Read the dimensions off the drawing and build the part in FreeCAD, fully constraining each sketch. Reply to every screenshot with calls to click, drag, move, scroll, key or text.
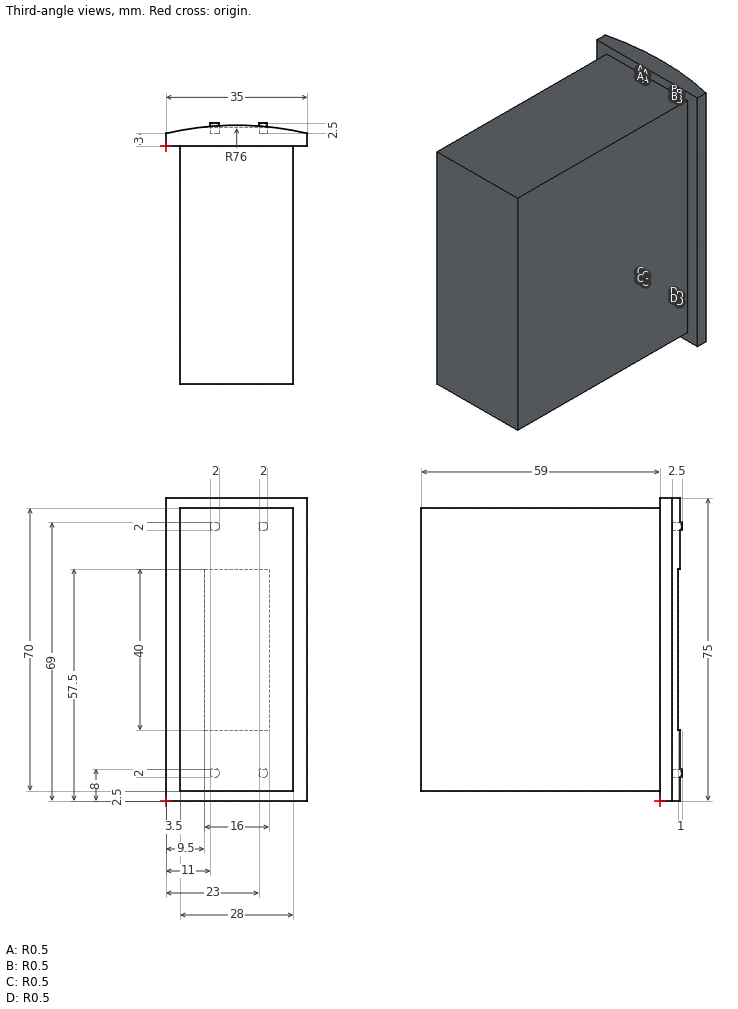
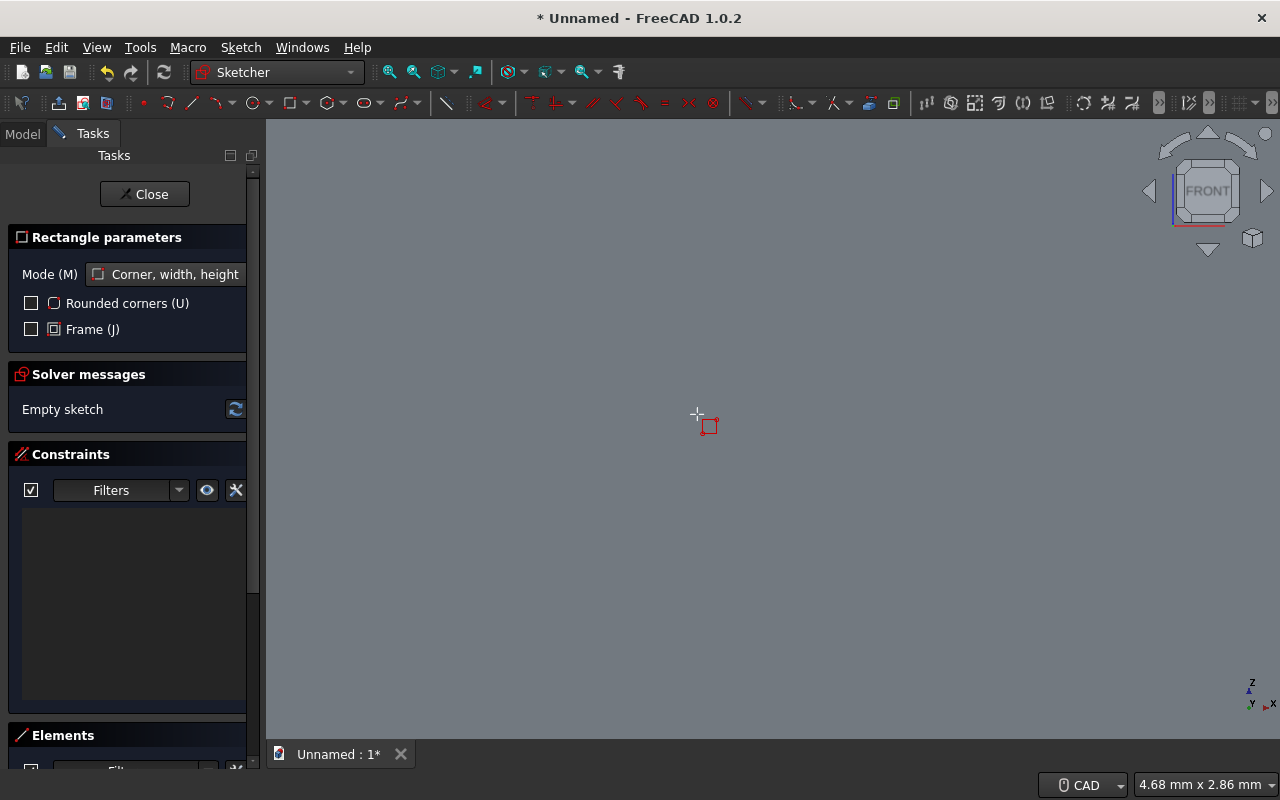
click(487, 212)
click(921, 645)
key(Escape)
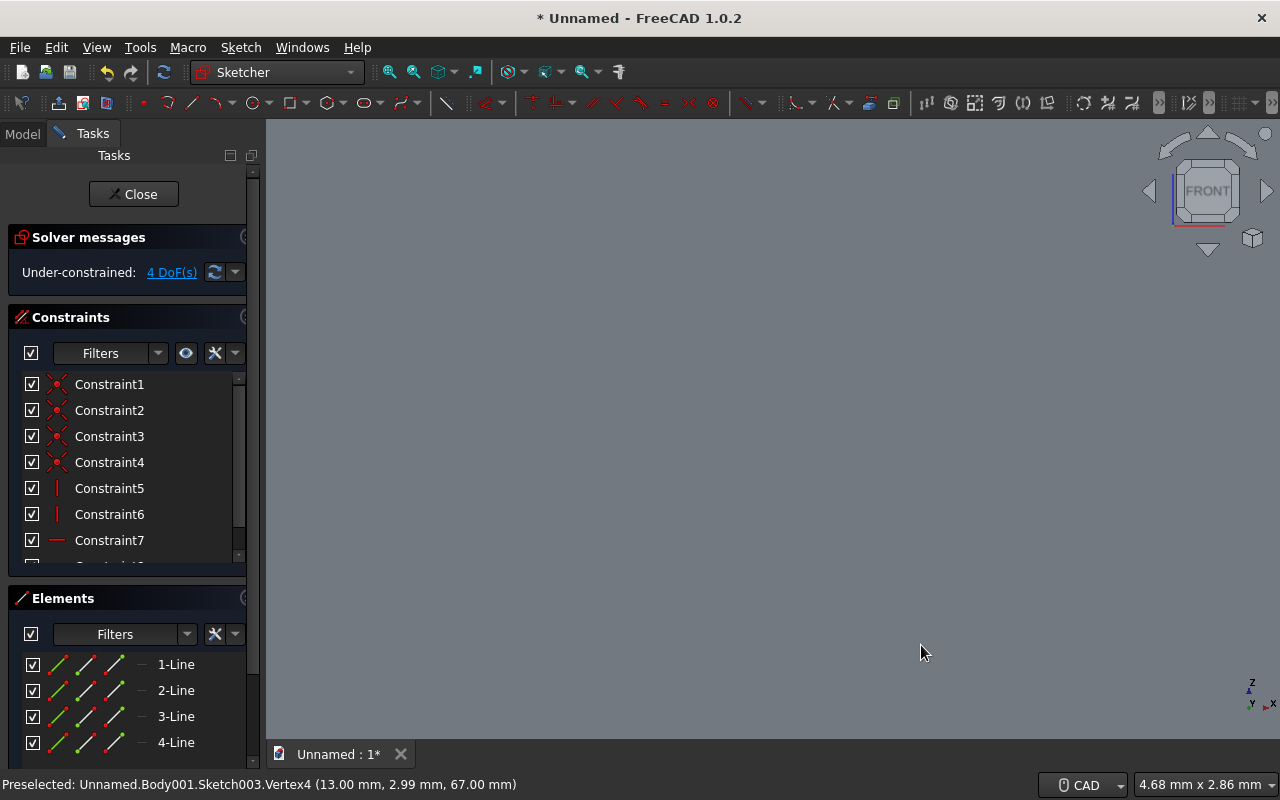
click(486, 104)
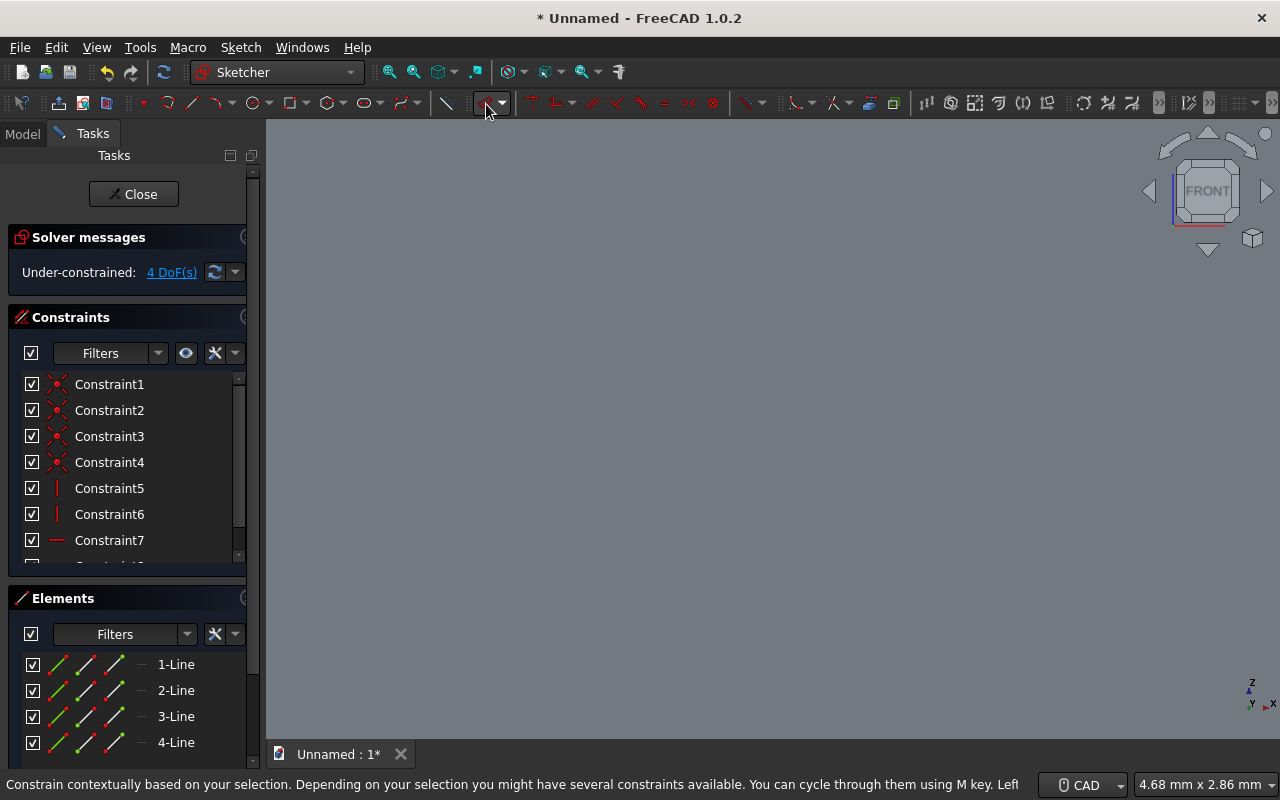
click(487, 343)
click(453, 430)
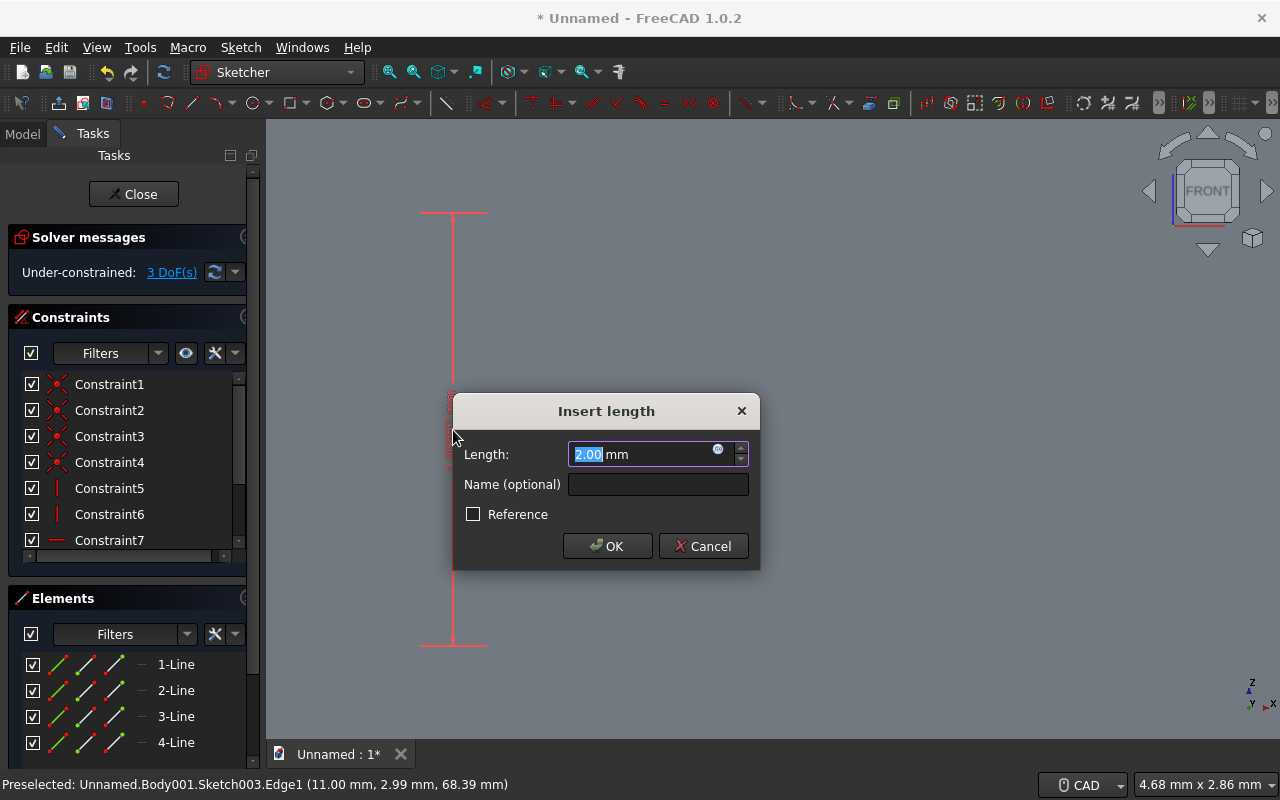
text(2)
key(Return)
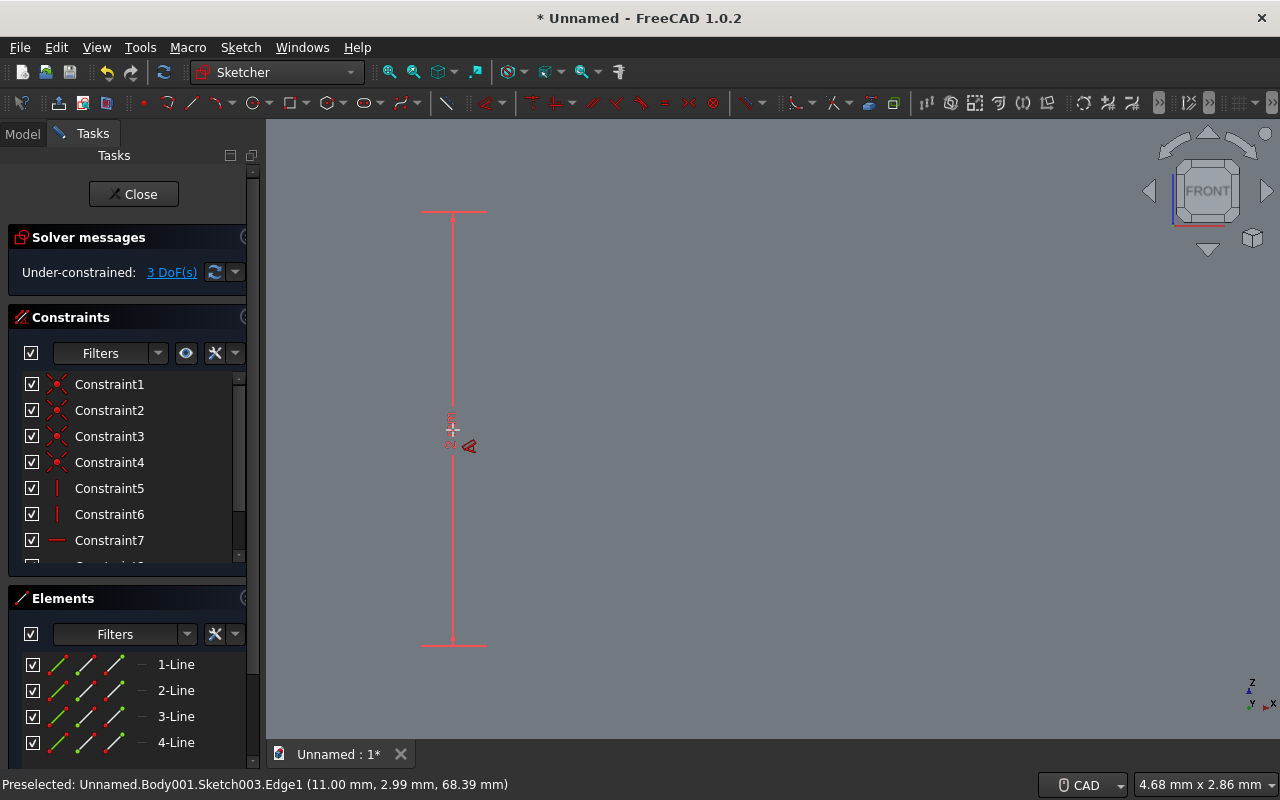
click(617, 646)
click(704, 680)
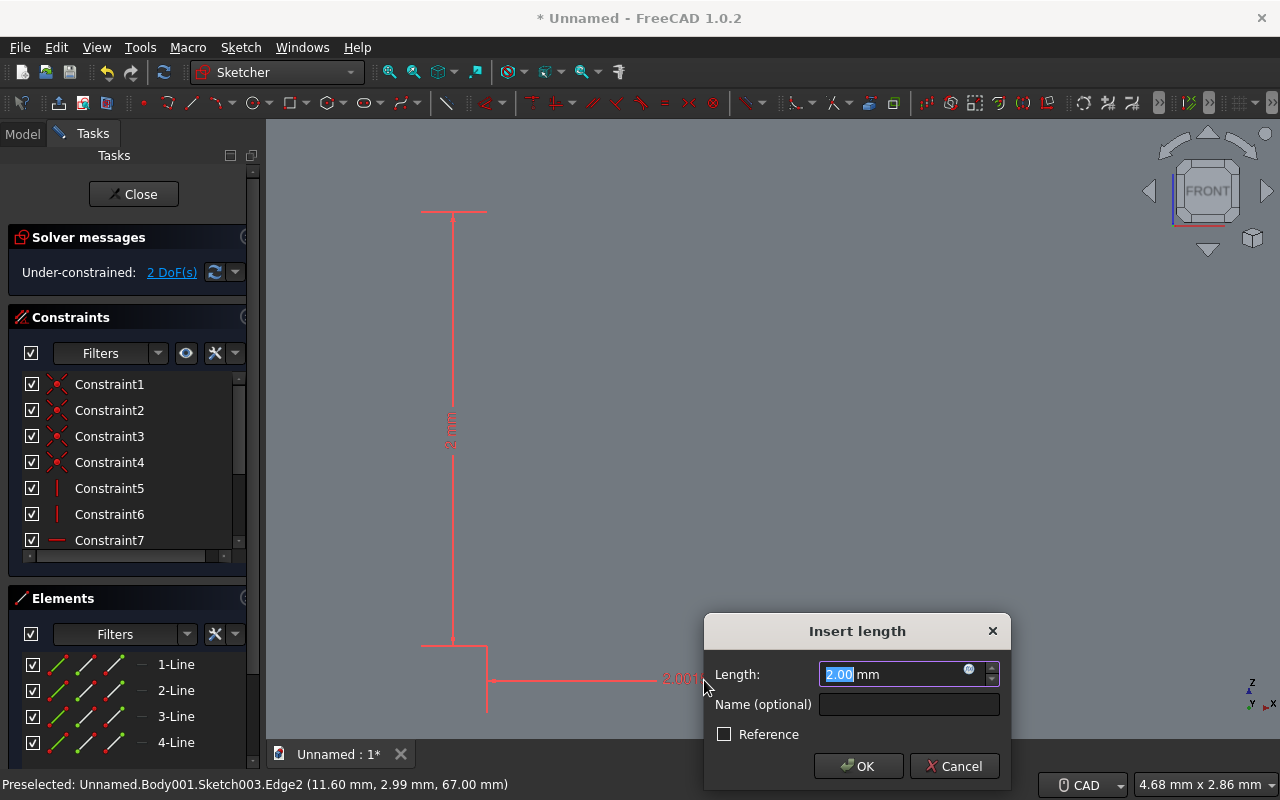
text(2)
key(Return)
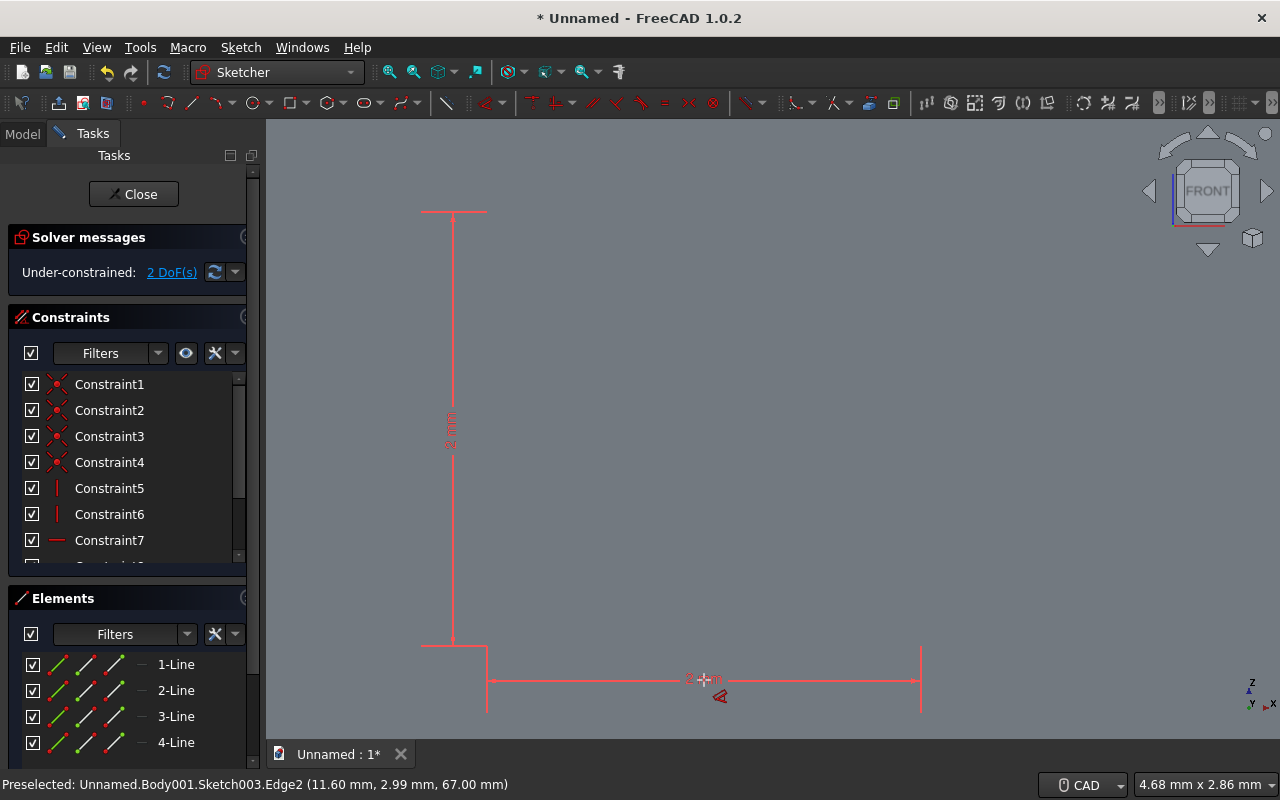
click(487, 212)
click(391, 178)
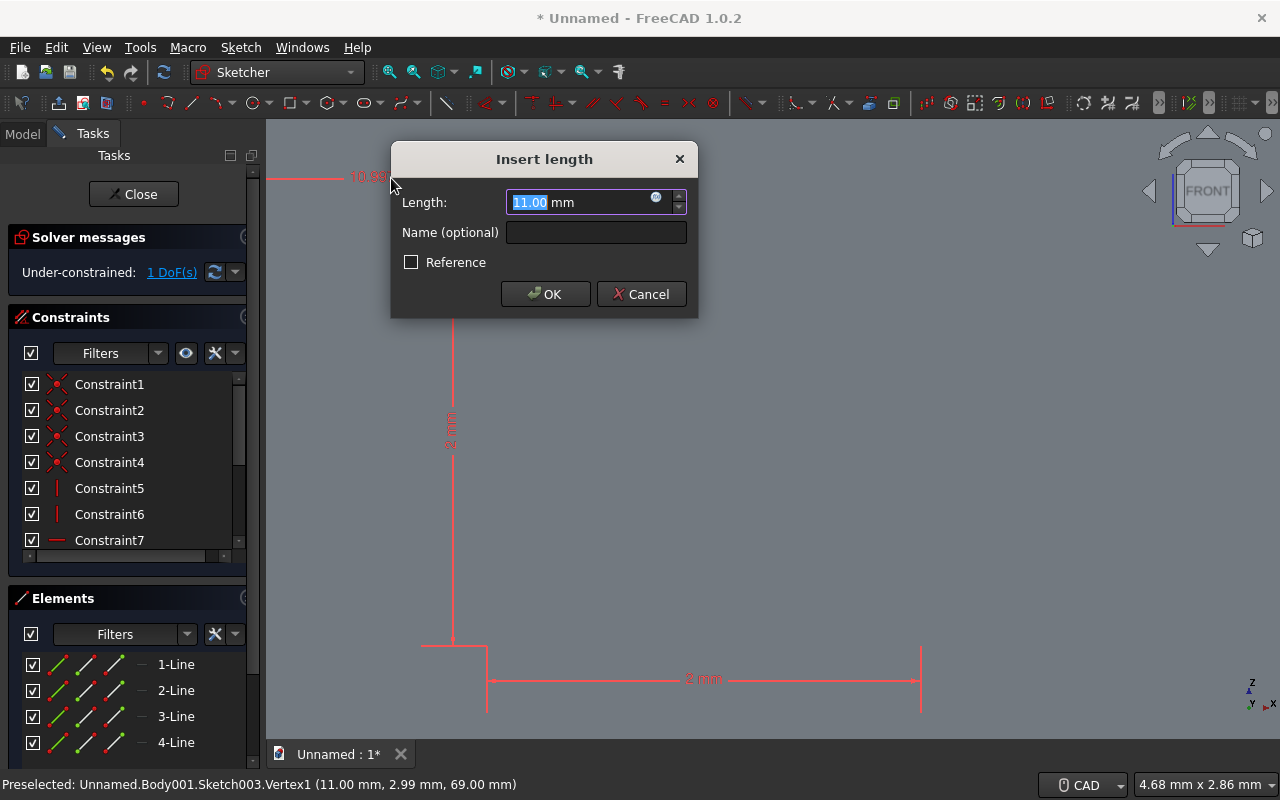
text(11)
key(Return)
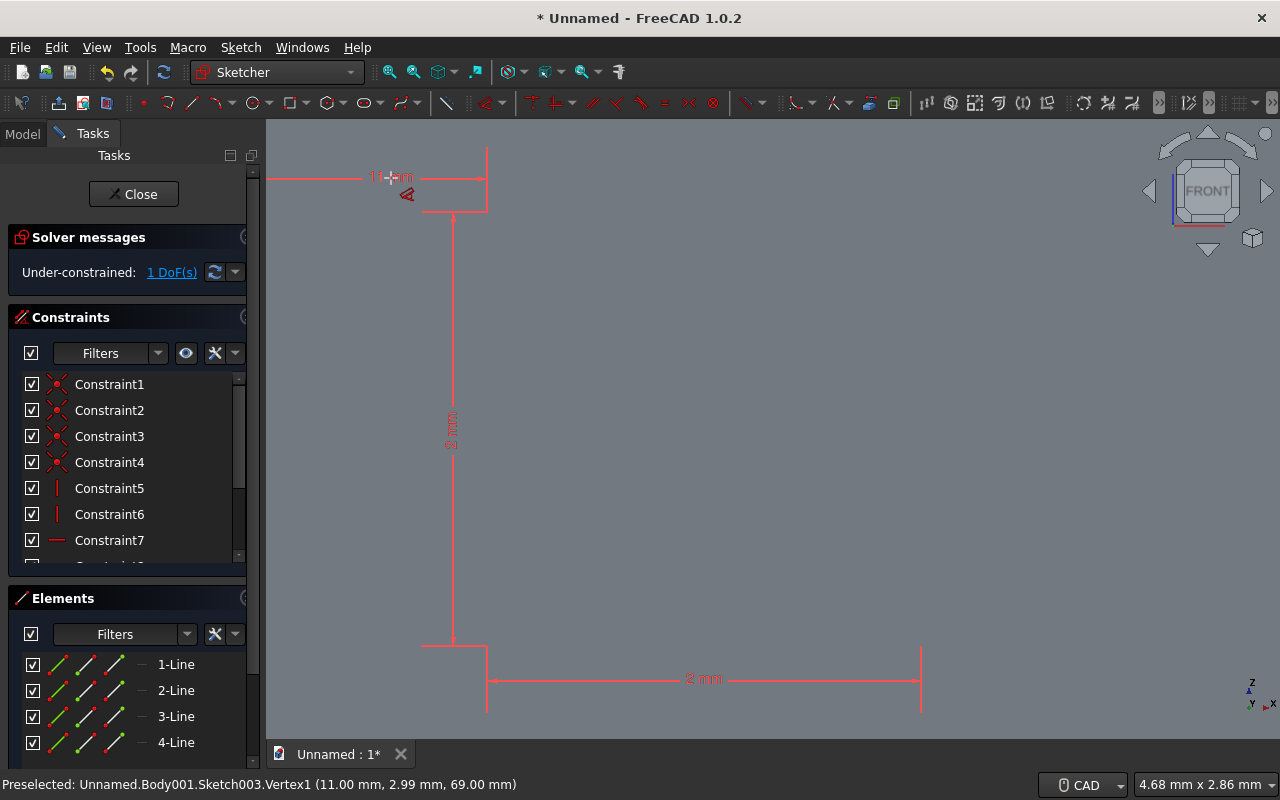
click(487, 212)
click(521, 462)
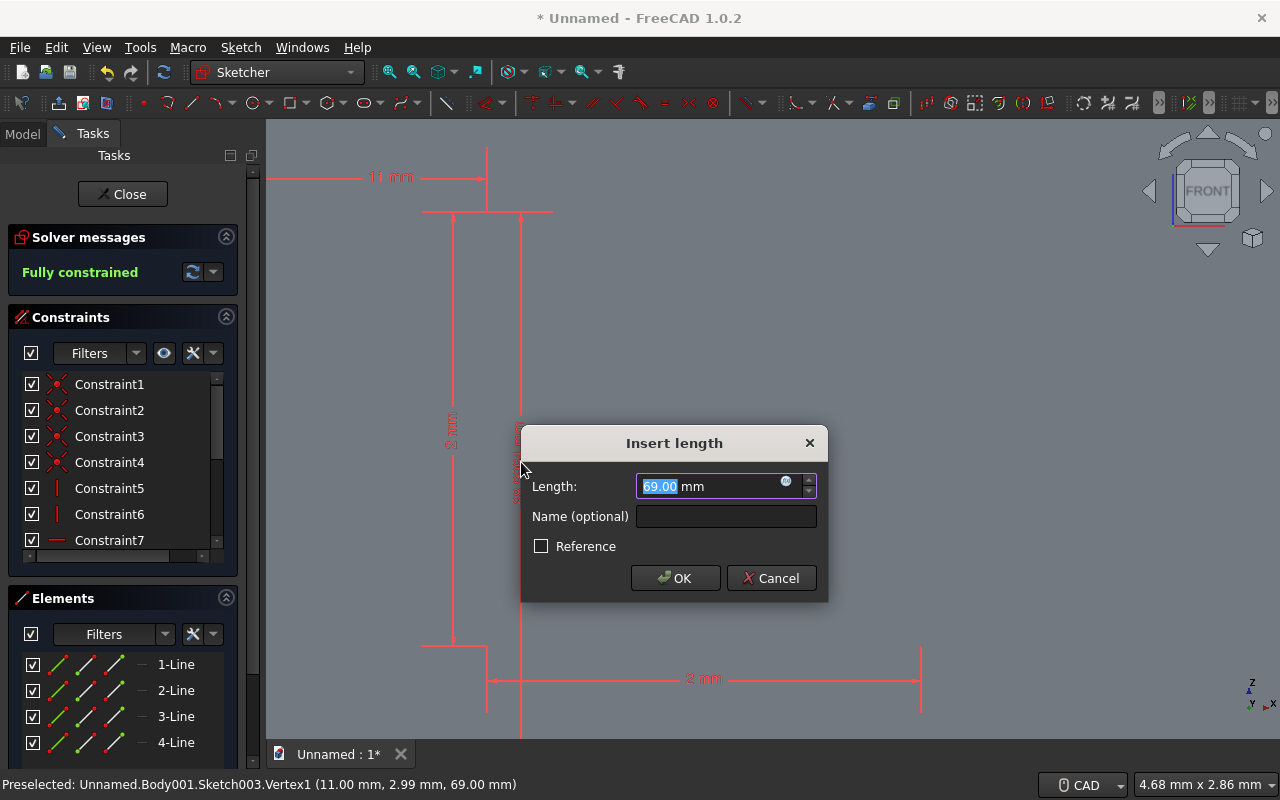
text(69)
key(Return)
key(Escape)